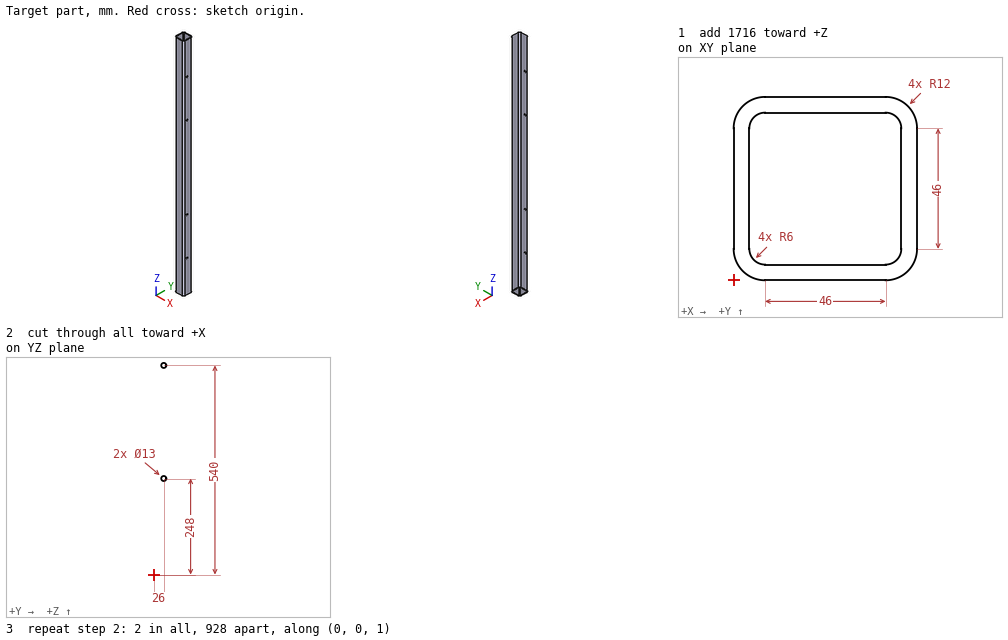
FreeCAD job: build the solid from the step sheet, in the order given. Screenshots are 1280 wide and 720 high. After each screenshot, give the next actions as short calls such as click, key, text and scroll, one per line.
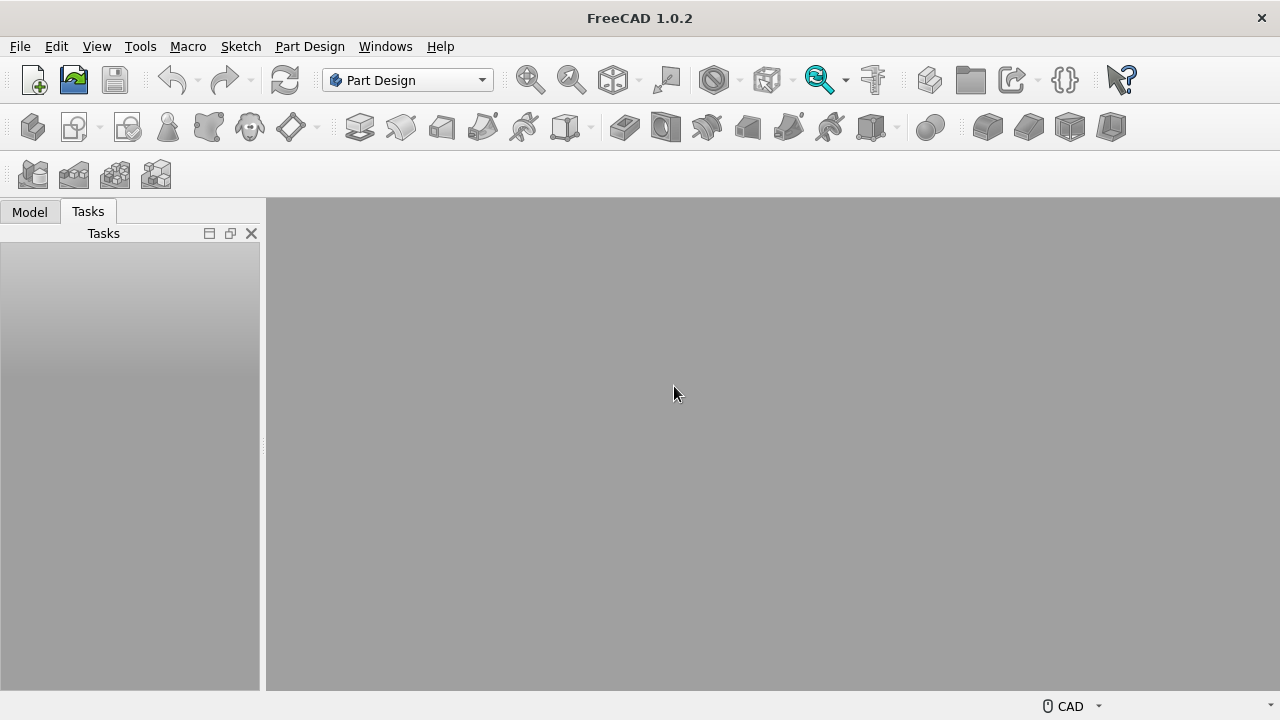
click(33, 80)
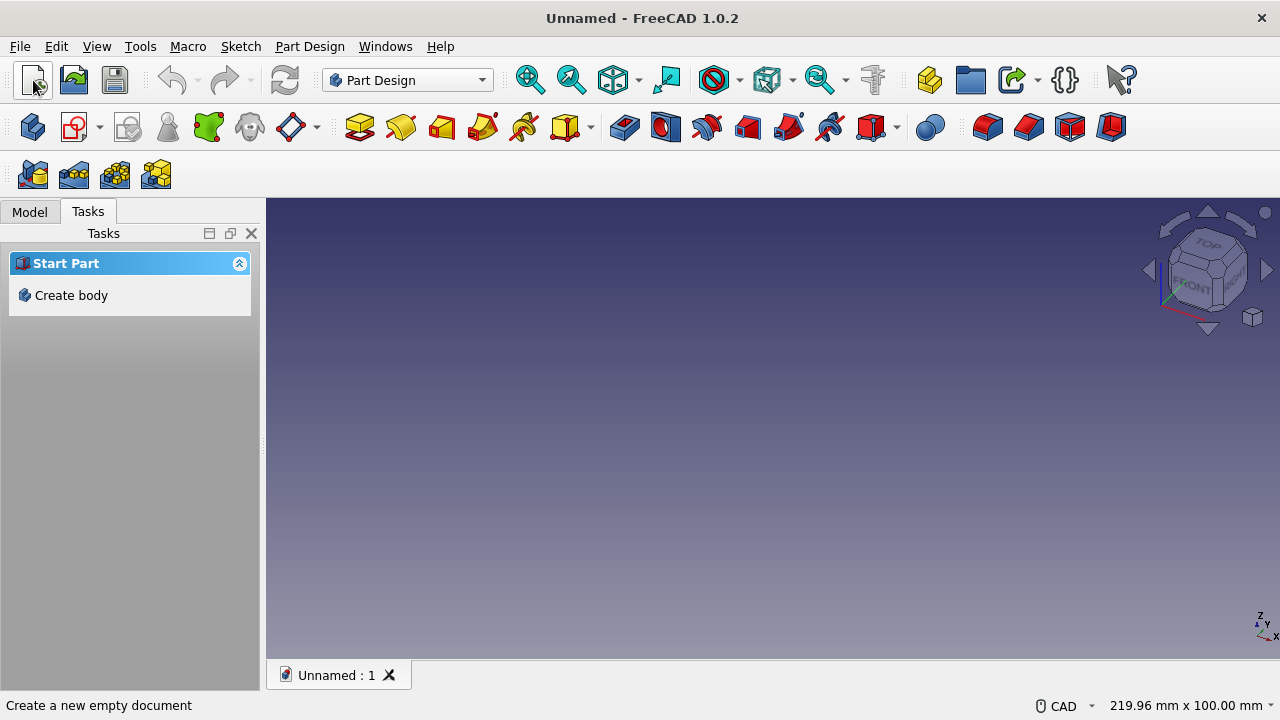
click(74, 128)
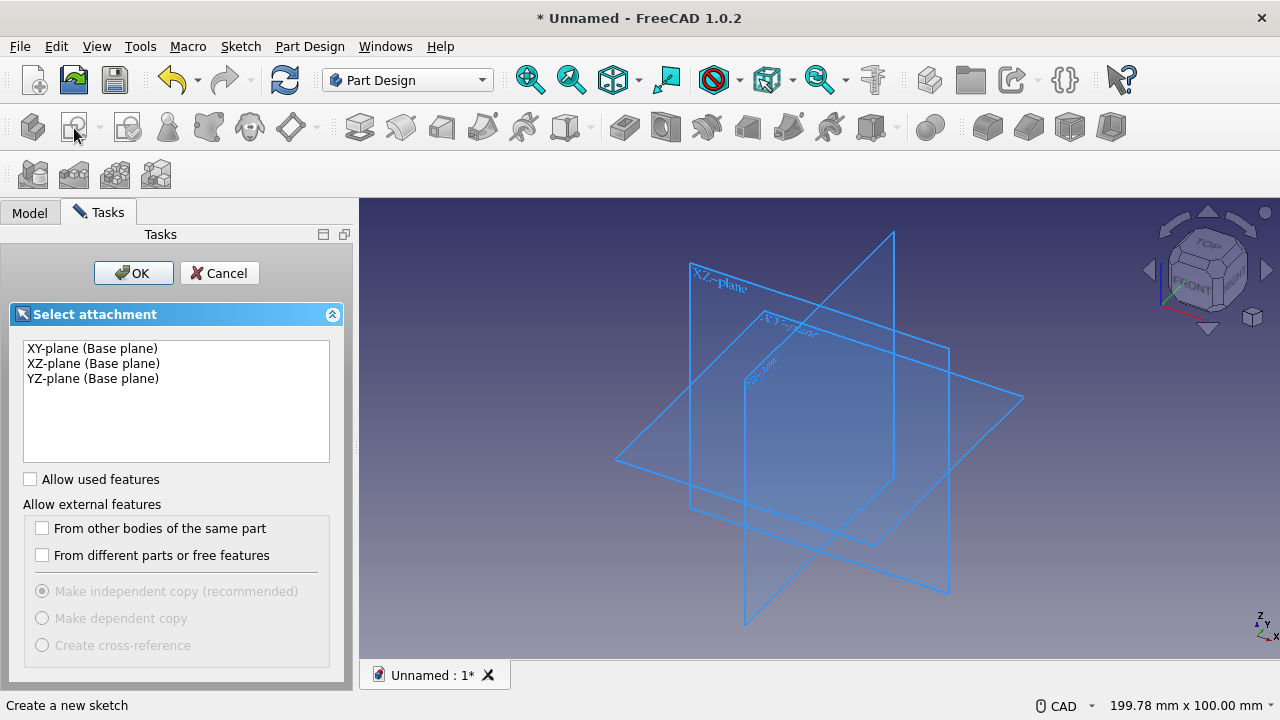
click(84, 348)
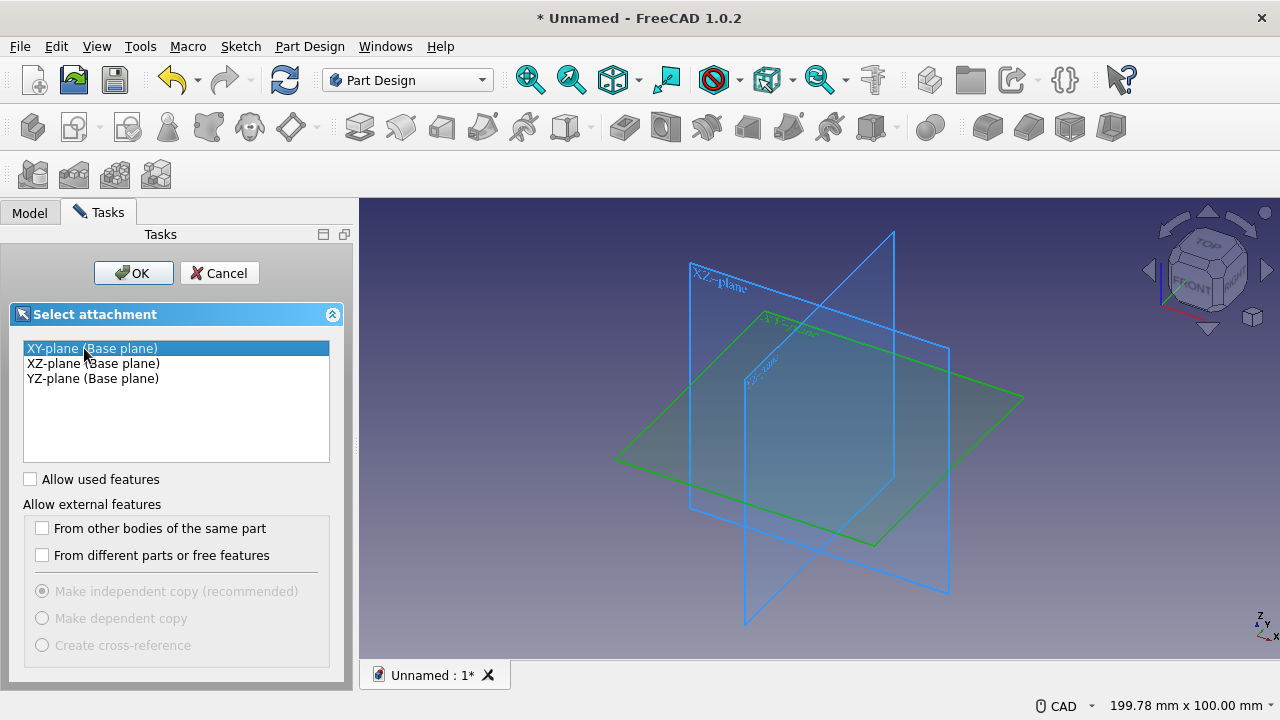
click(134, 273)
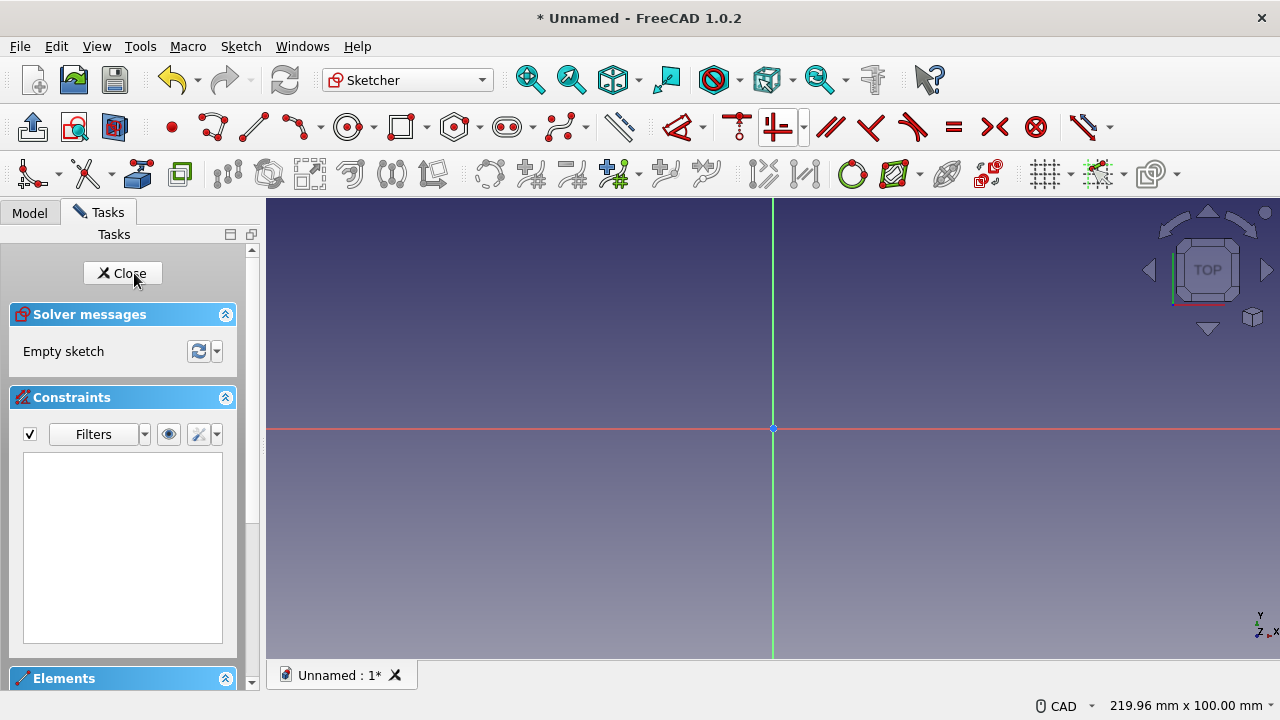
scroll(294, 631, down, 2)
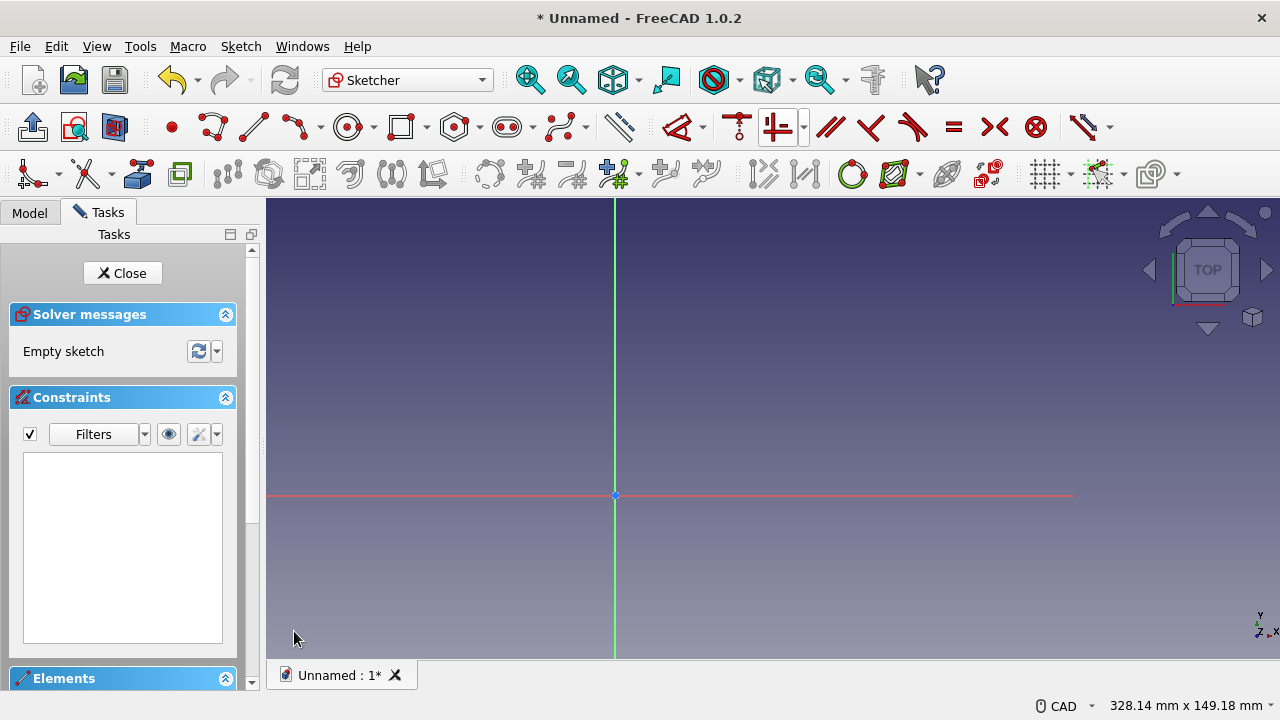
click(254, 128)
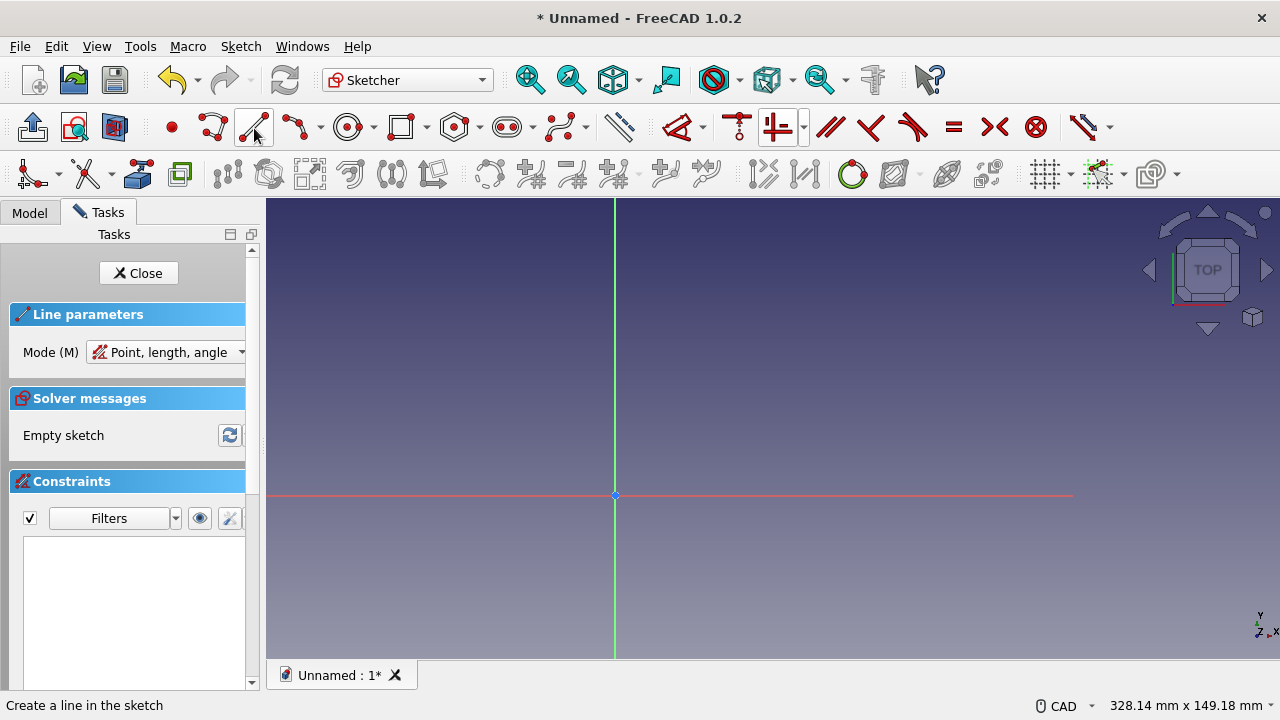
click(652, 496)
click(794, 487)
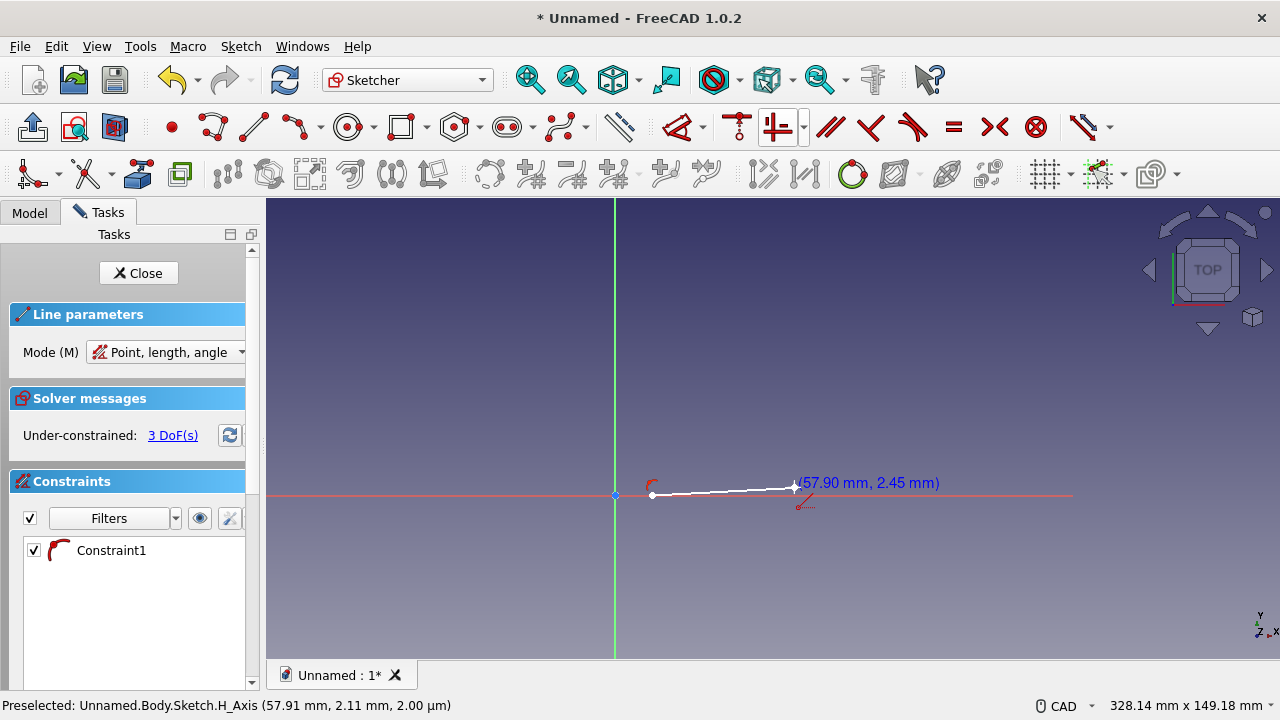
click(831, 458)
click(831, 316)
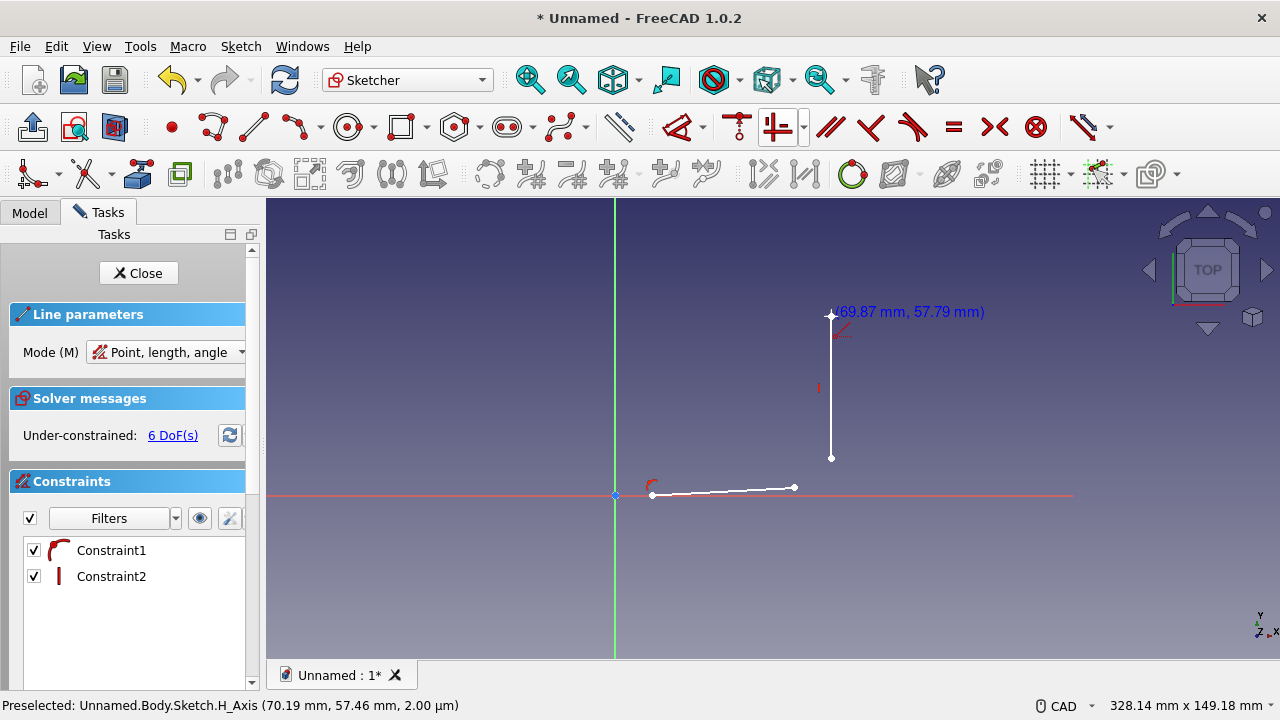
click(794, 279)
click(652, 279)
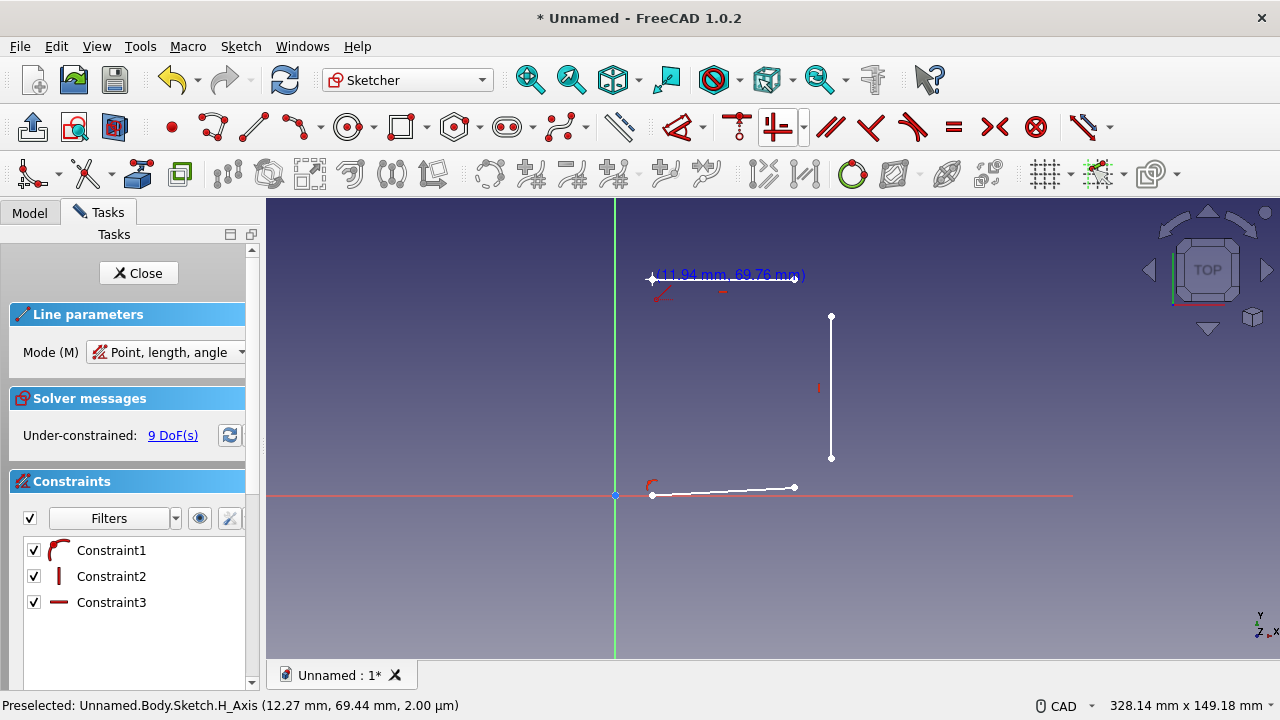
click(615, 316)
click(624, 458)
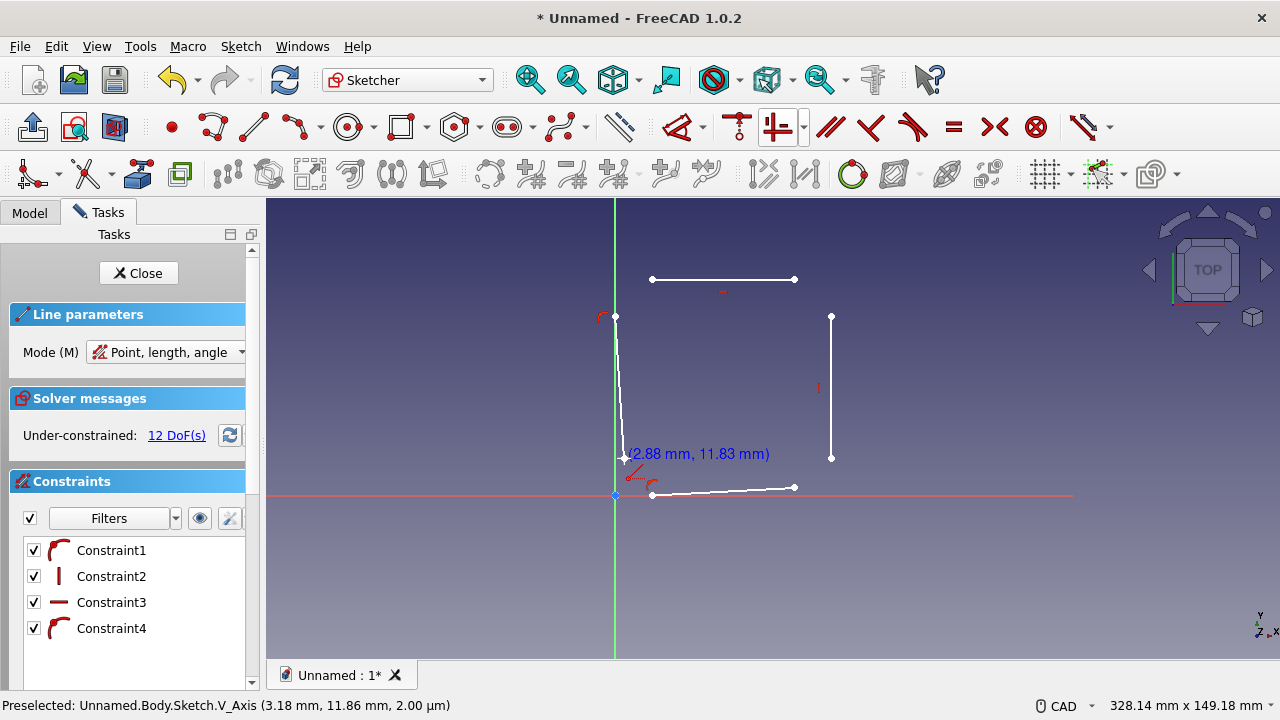
click(294, 128)